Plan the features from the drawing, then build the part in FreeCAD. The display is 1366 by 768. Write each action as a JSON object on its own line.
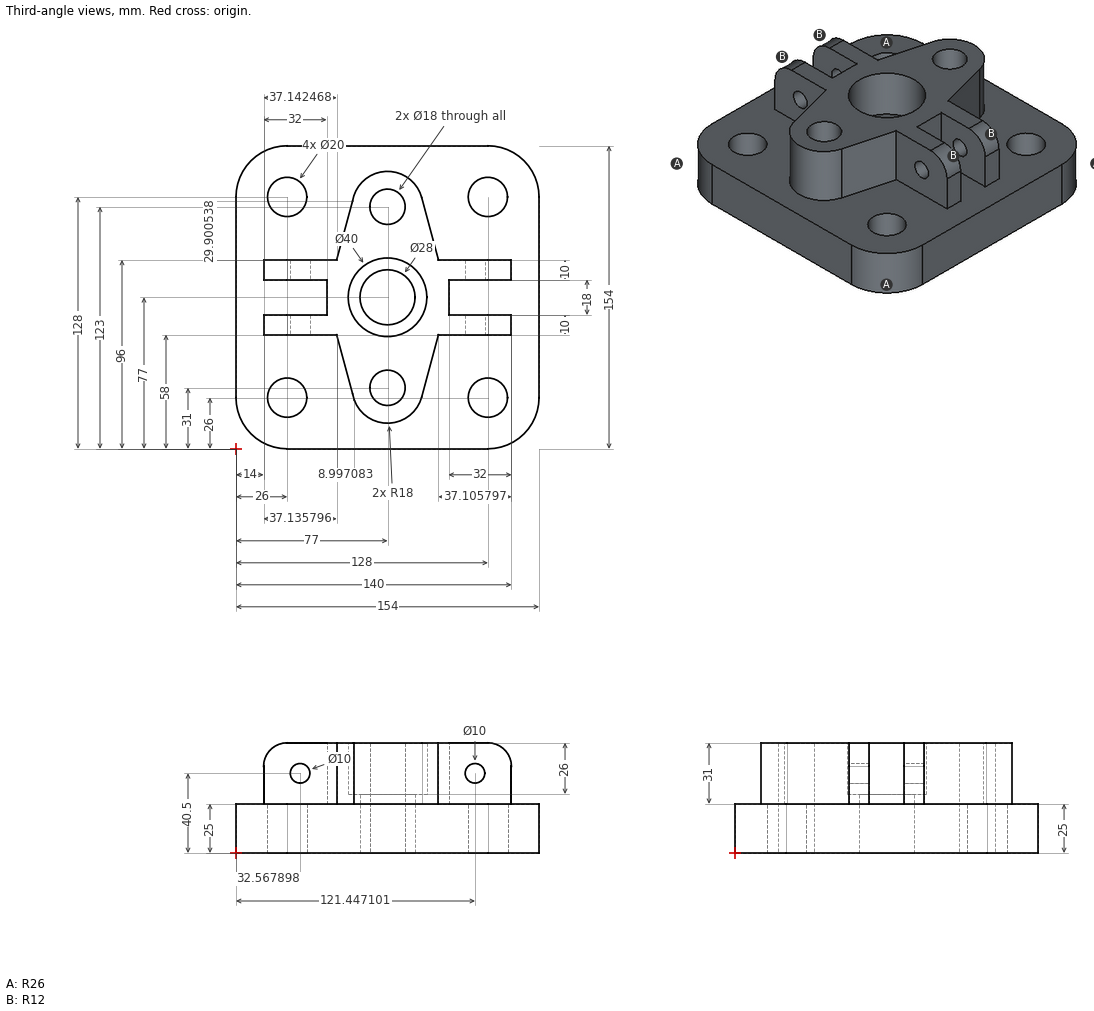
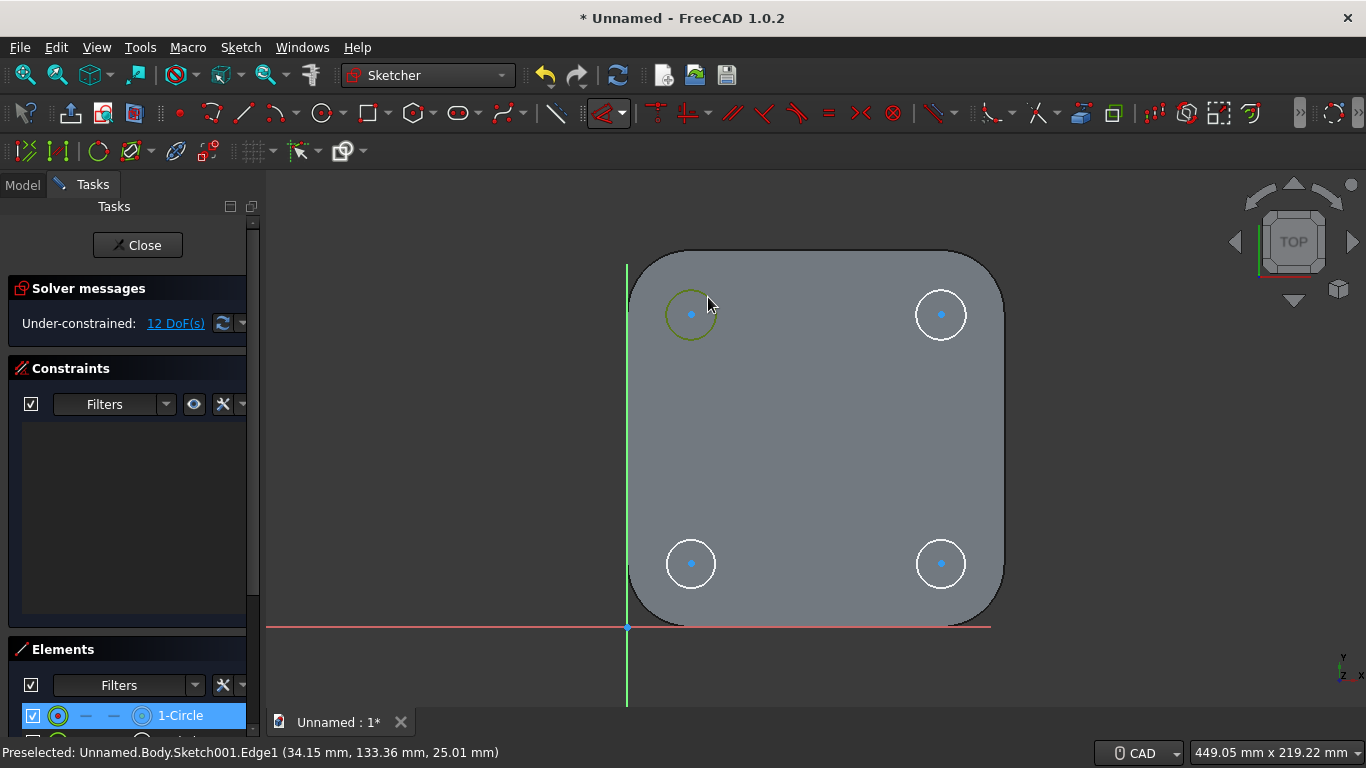
{"action": "left_click", "coordinate": [958, 297]}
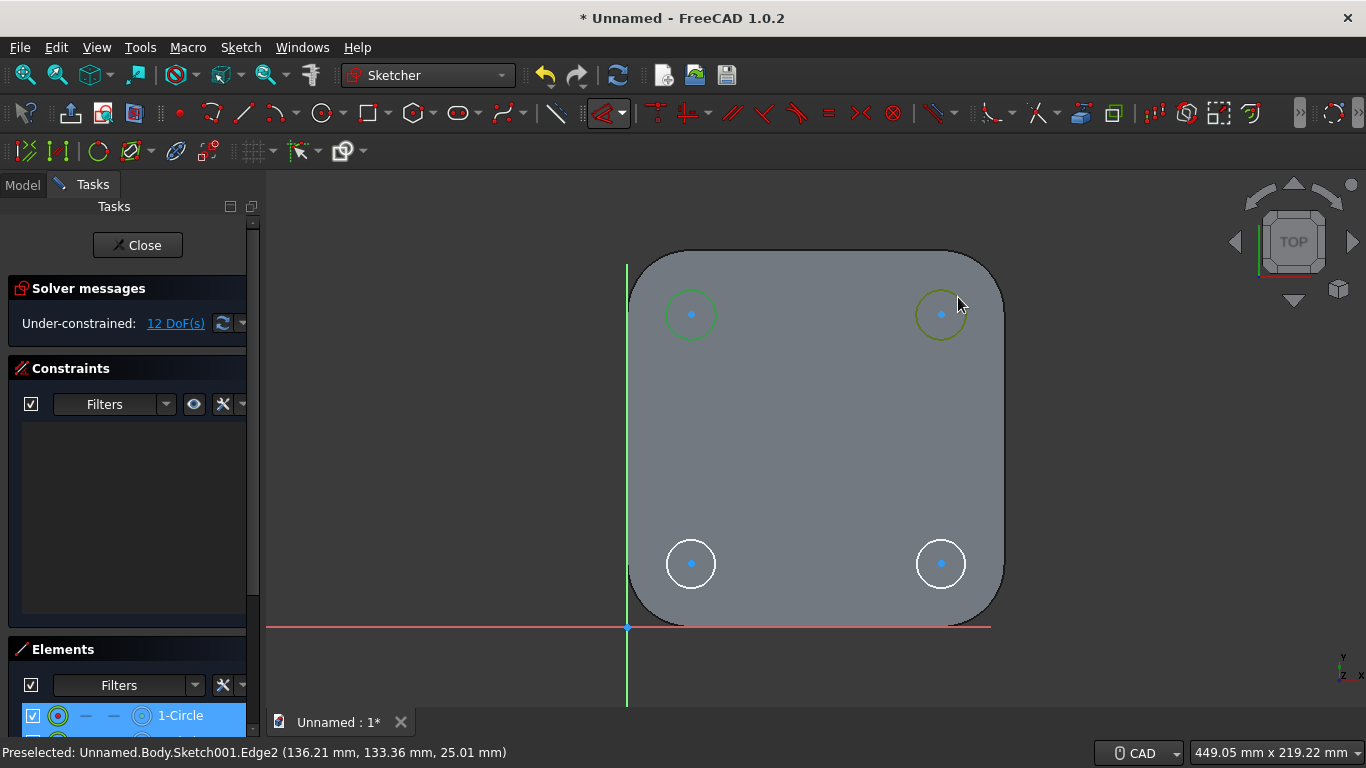
{"action": "left_click", "coordinate": [958, 547]}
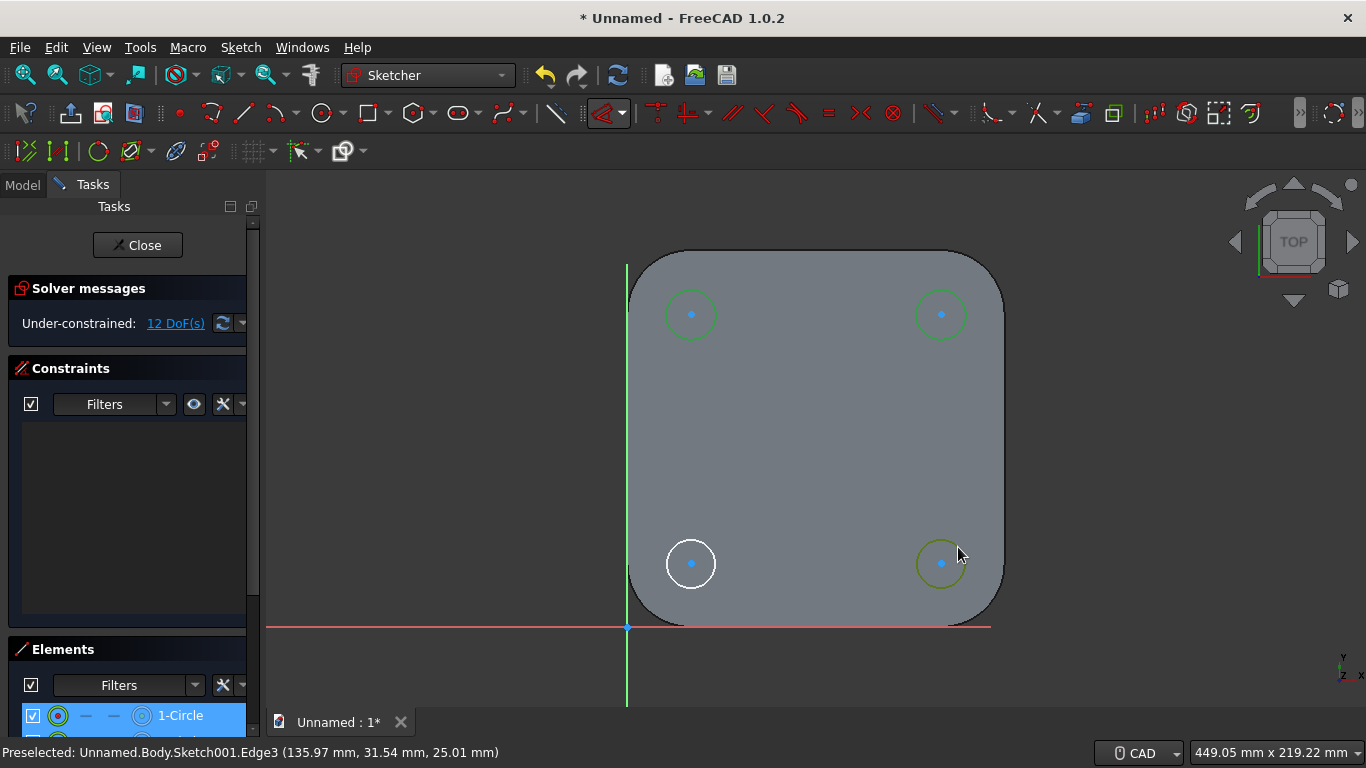
{"action": "left_click", "coordinate": [708, 547]}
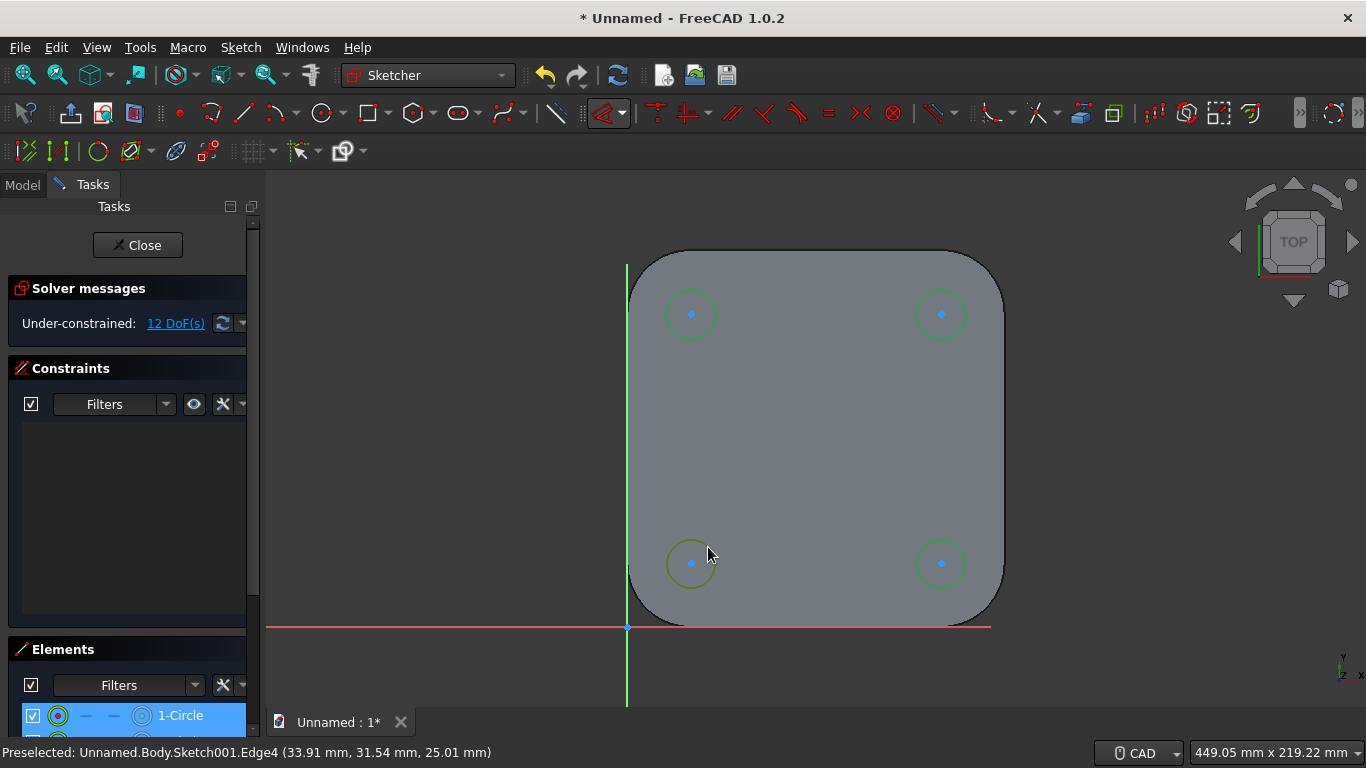
{"action": "left_click", "coordinate": [830, 114]}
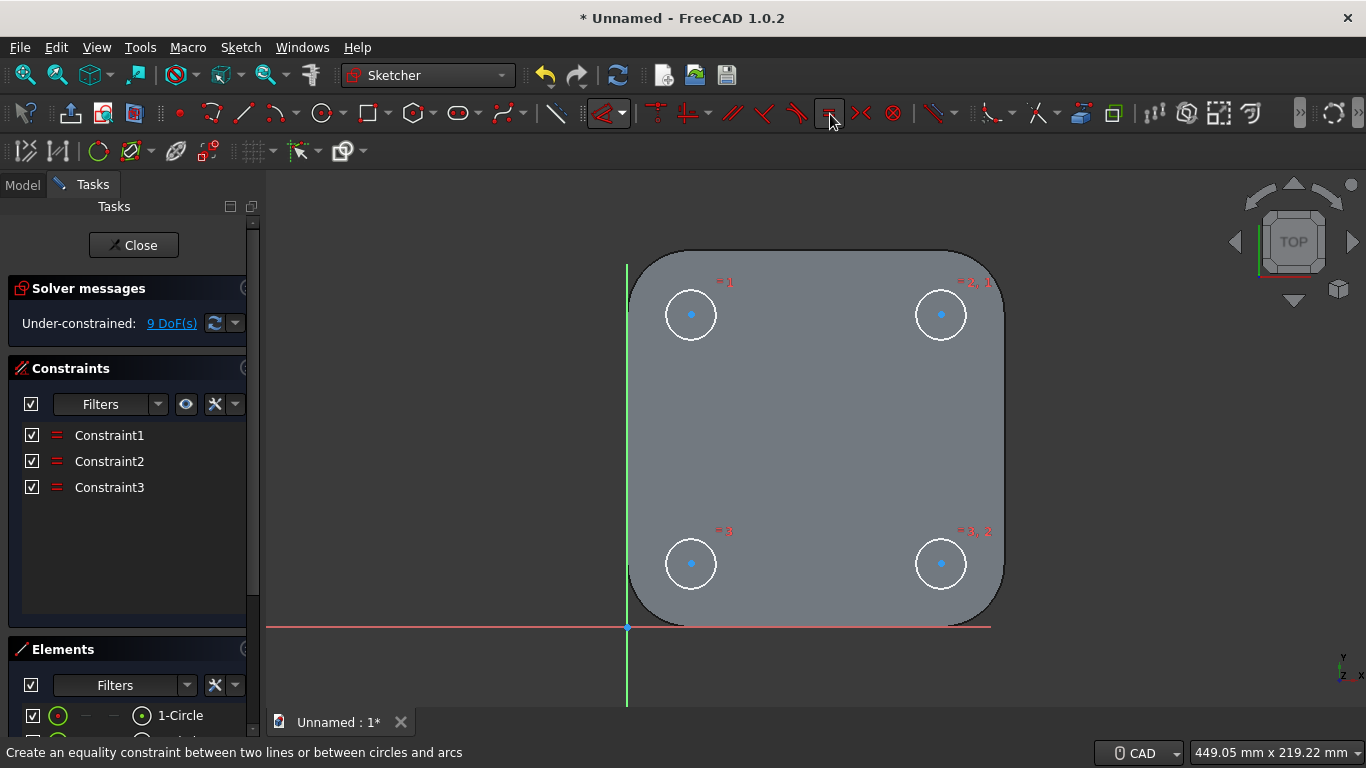
{"action": "left_click", "coordinate": [708, 297]}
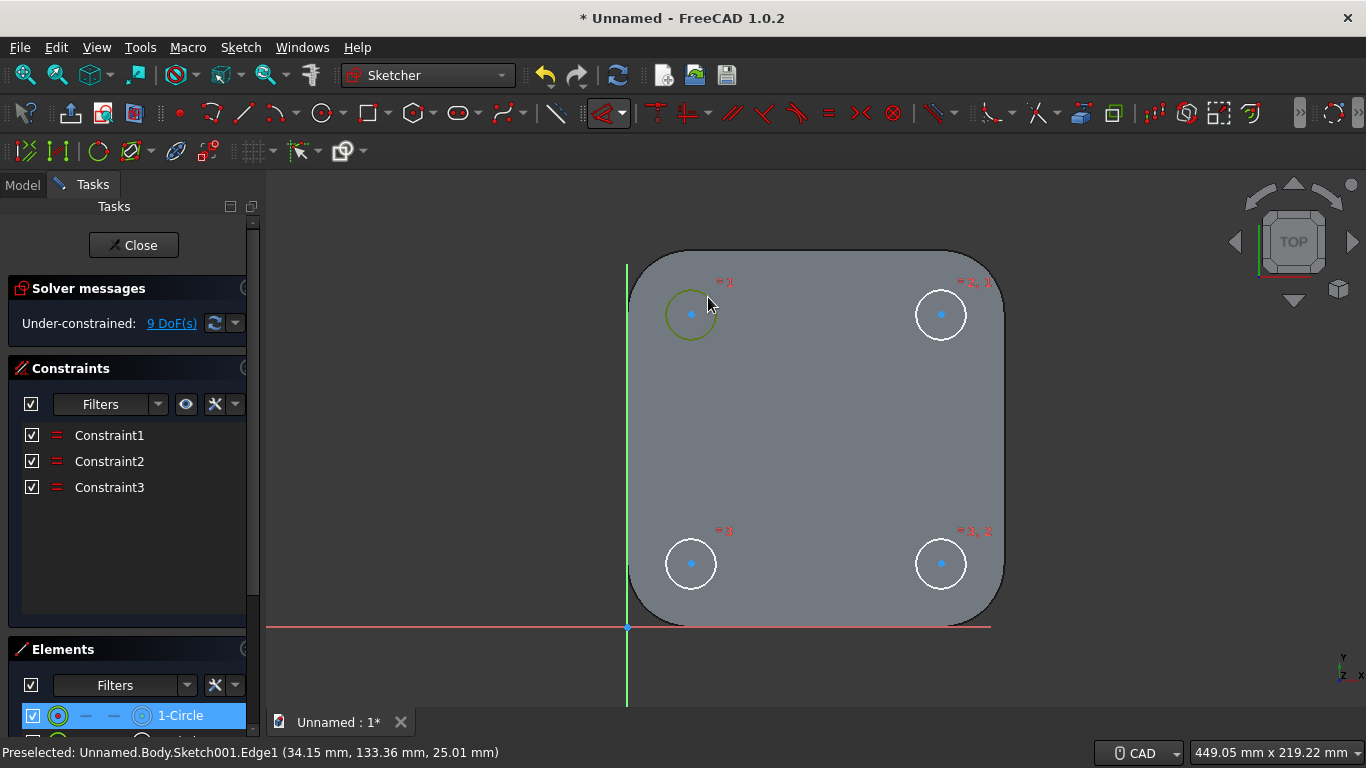
{"action": "left_click", "coordinate": [624, 114]}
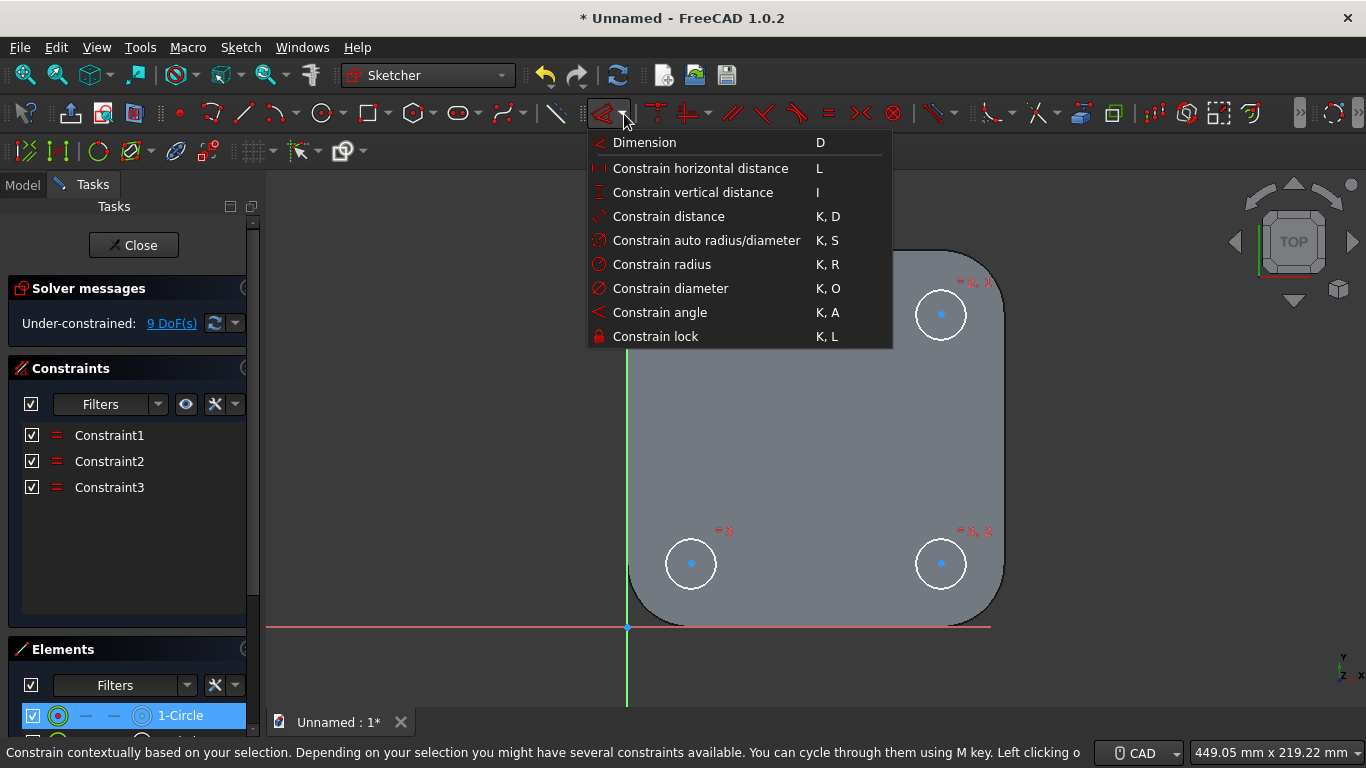
{"action": "left_click", "coordinate": [740, 288]}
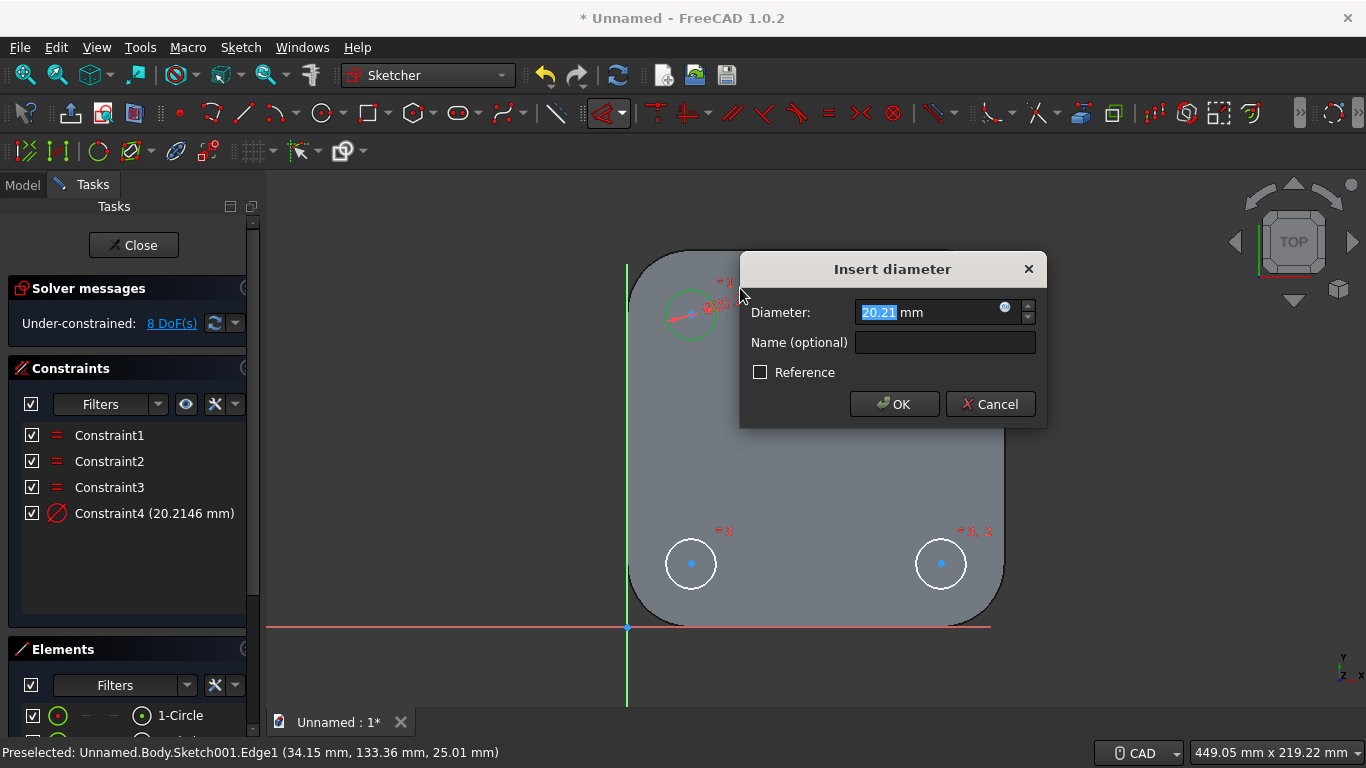
{"action": "type", "text": "20"}
{"action": "key", "text": "Return"}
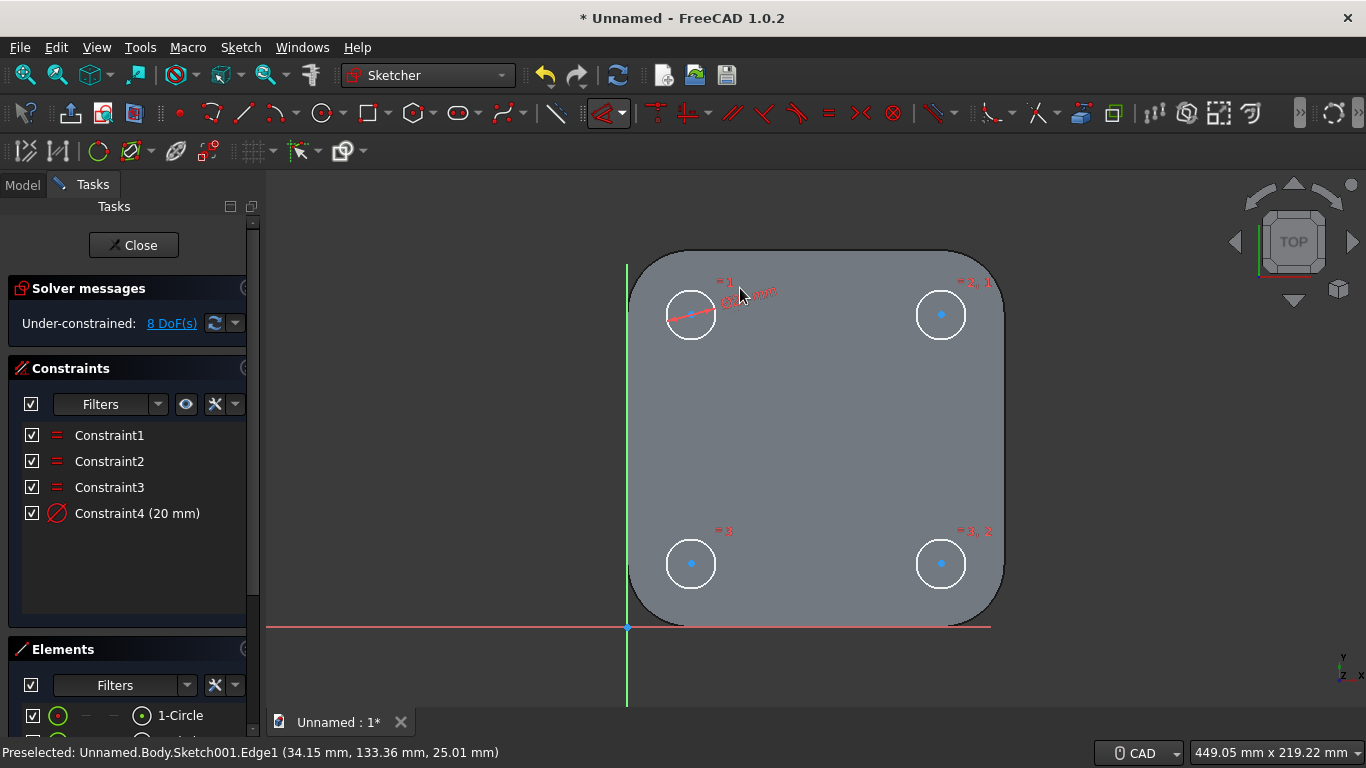
{"action": "left_click", "coordinate": [691, 315]}